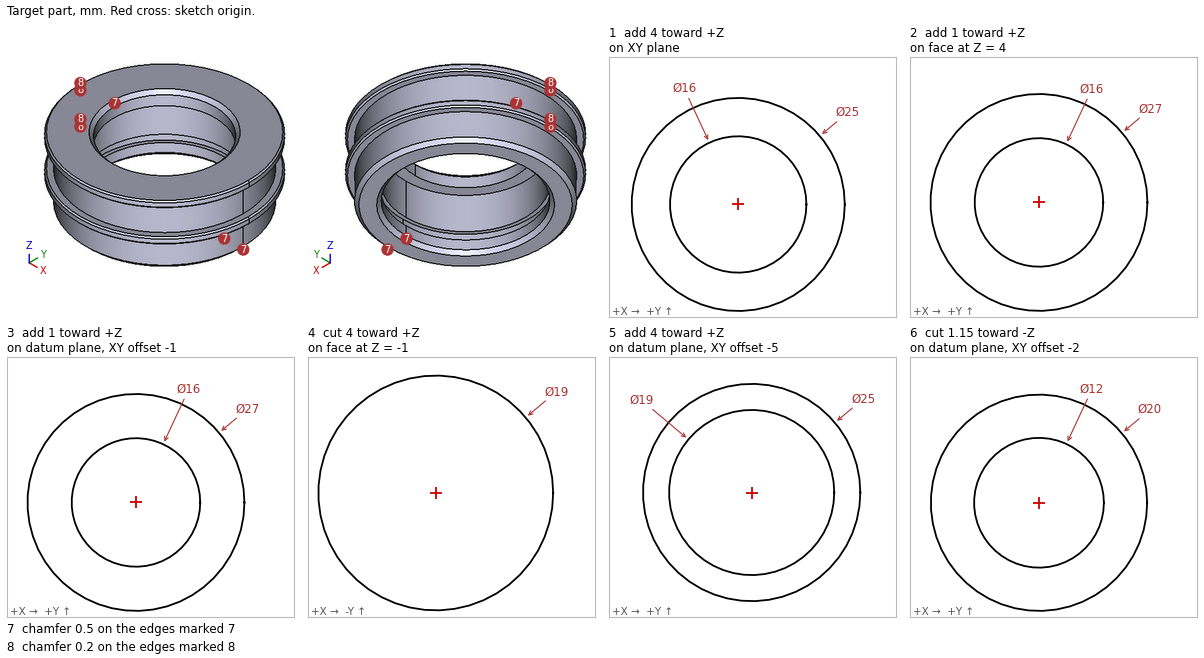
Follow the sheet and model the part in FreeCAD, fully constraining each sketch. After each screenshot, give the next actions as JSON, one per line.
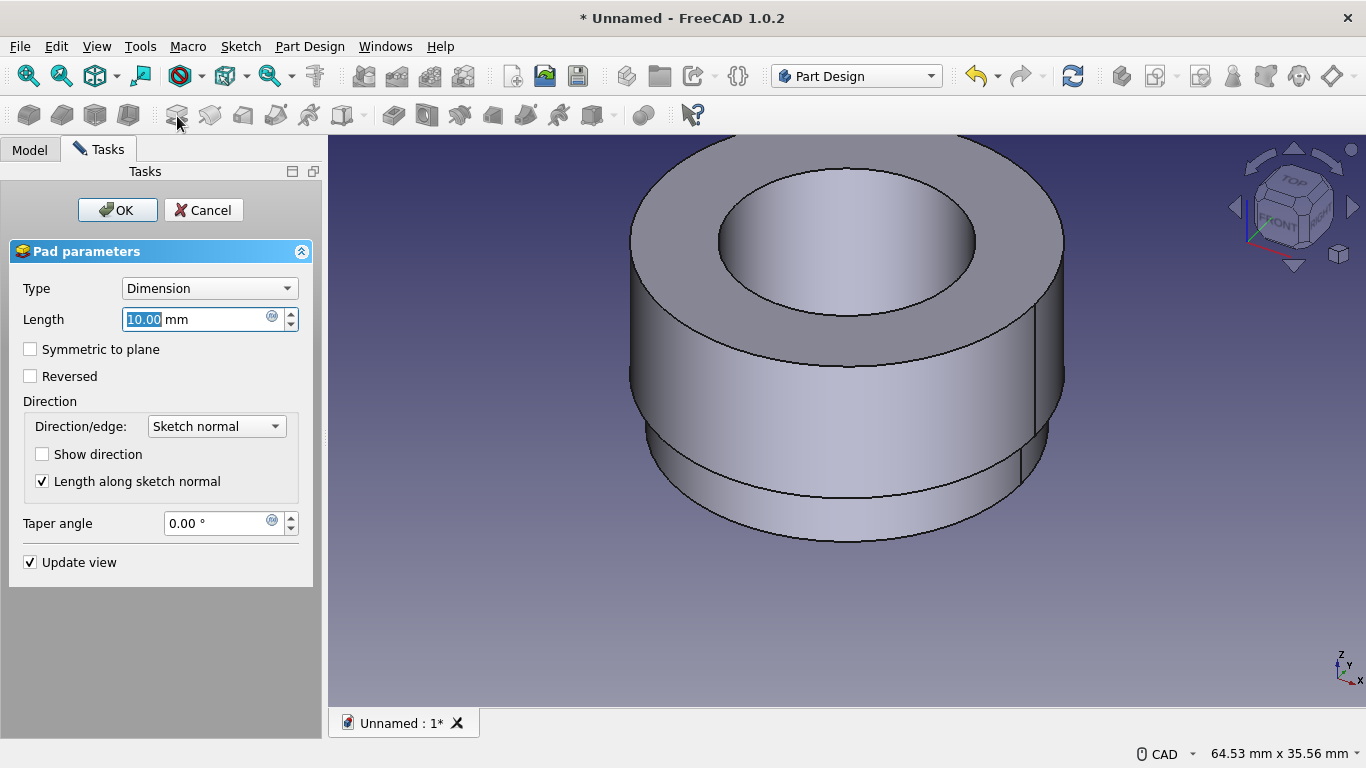
{"action": "type", "text": "1"}
{"action": "key", "text": "Tab"}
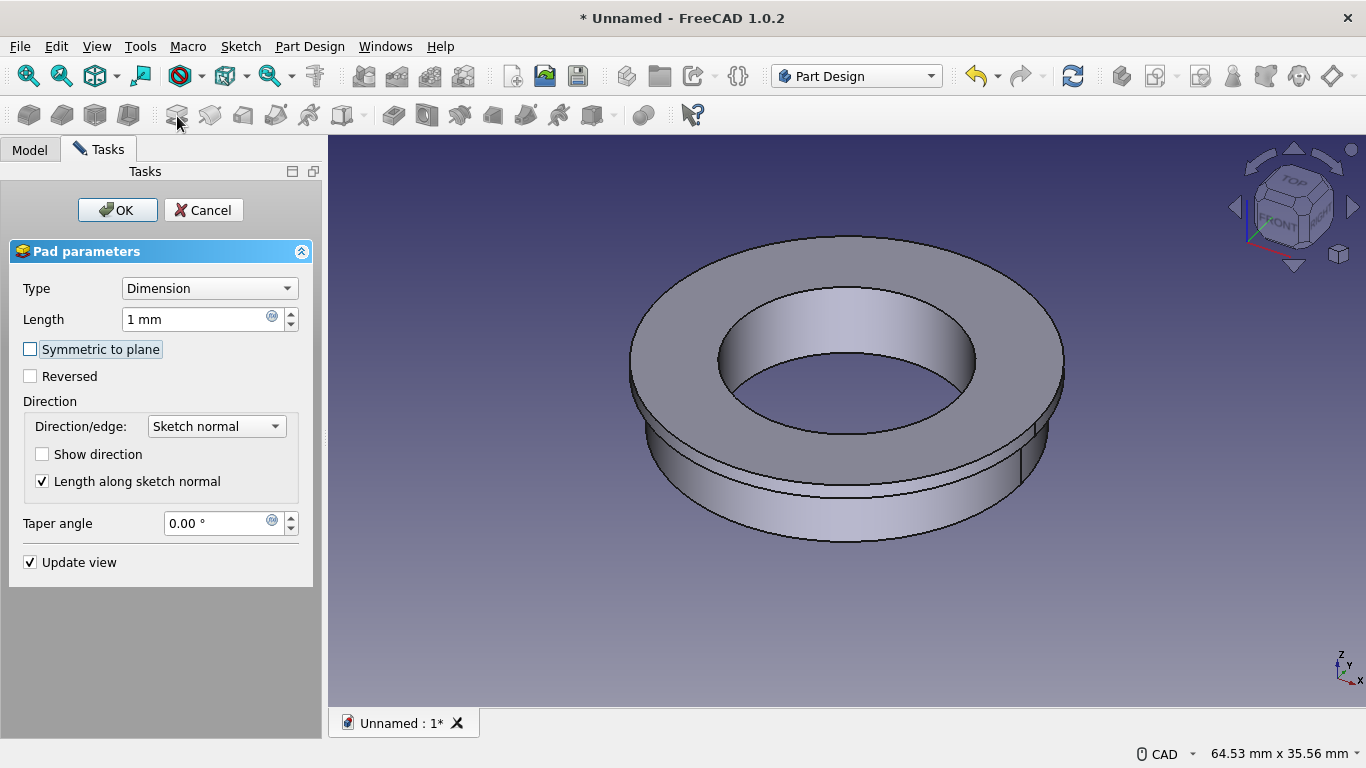
{"action": "left_click", "coordinate": [118, 210]}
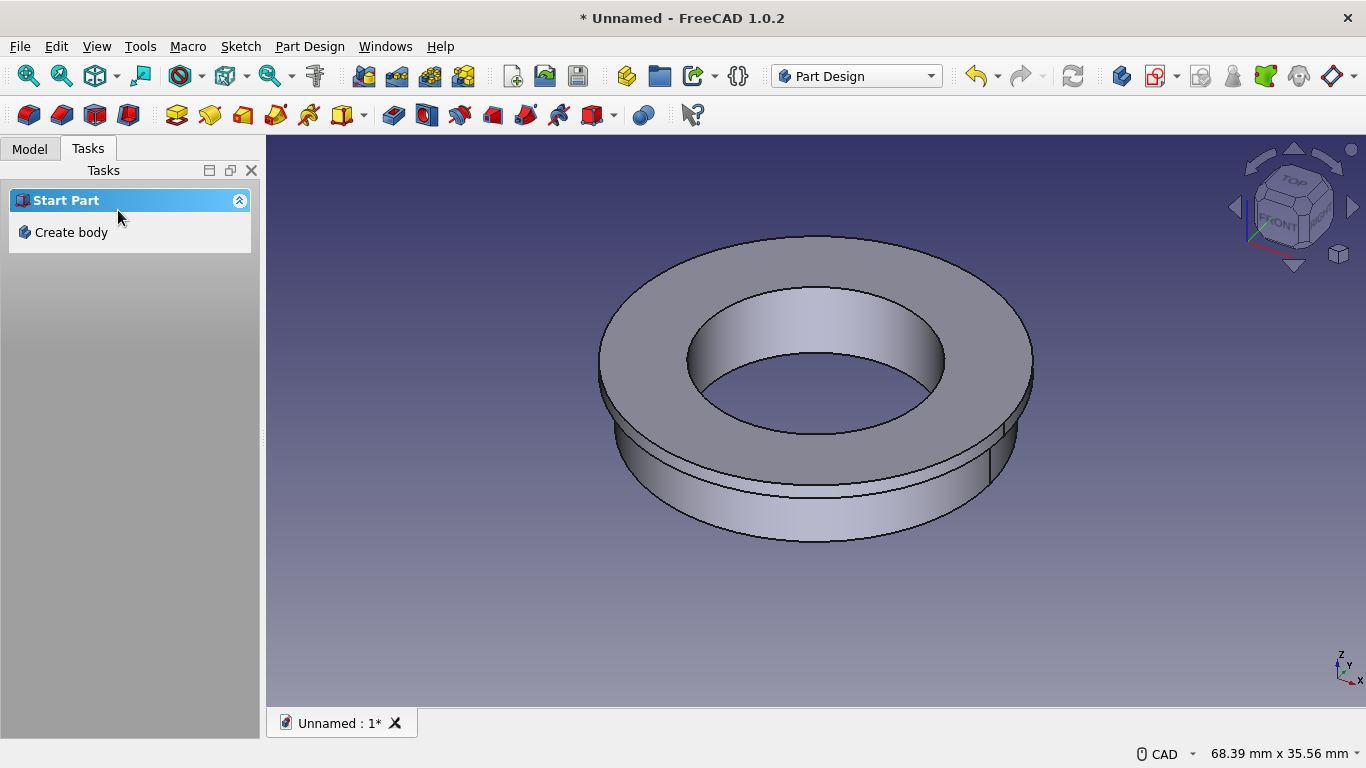
{"action": "left_click", "coordinate": [30, 148]}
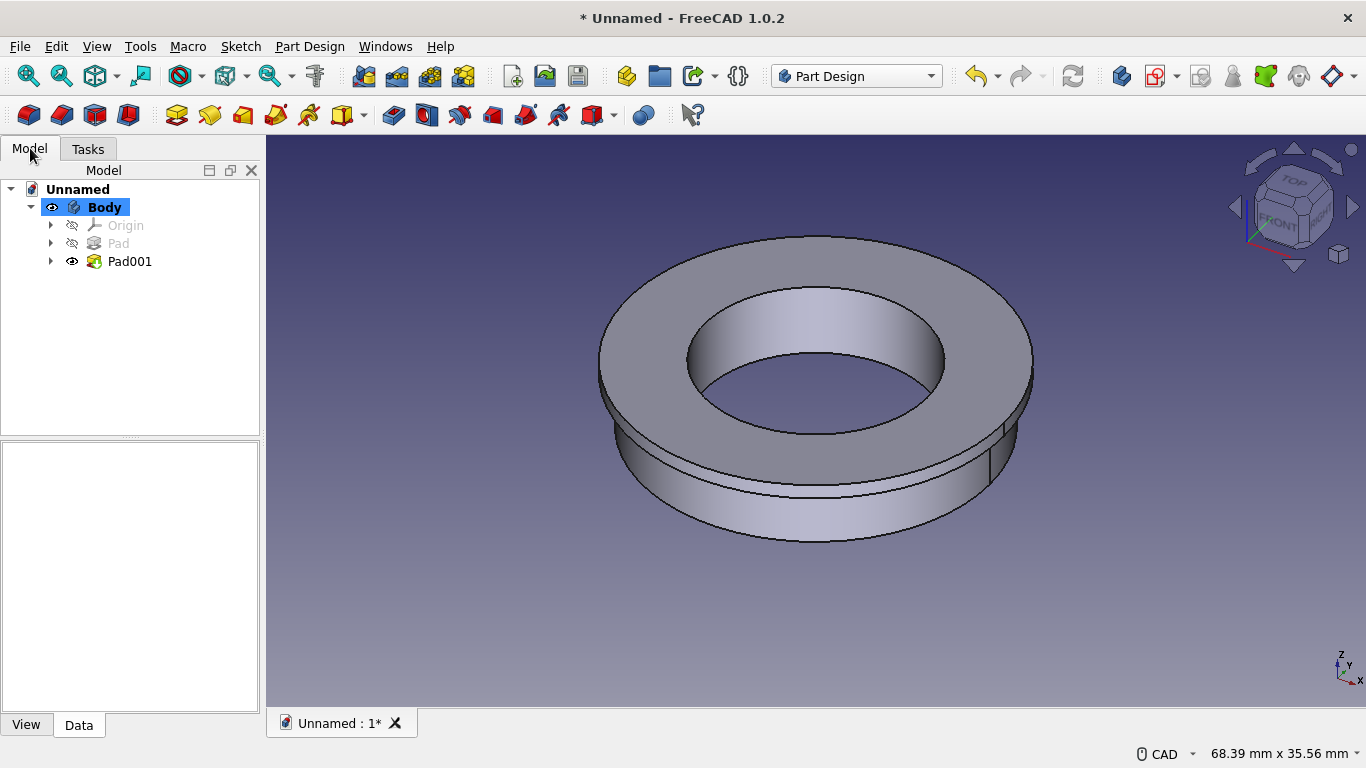
{"action": "left_click", "coordinate": [51, 225]}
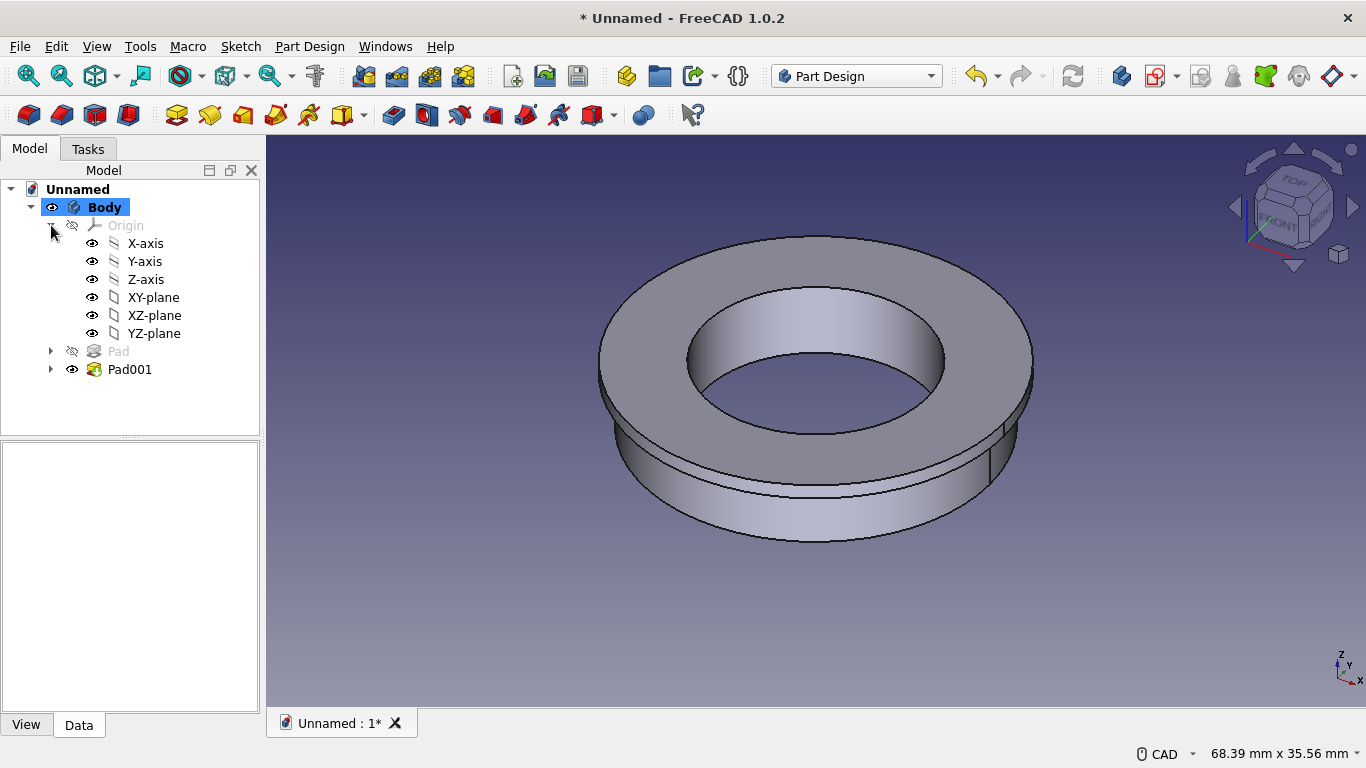
{"action": "left_click", "coordinate": [137, 297]}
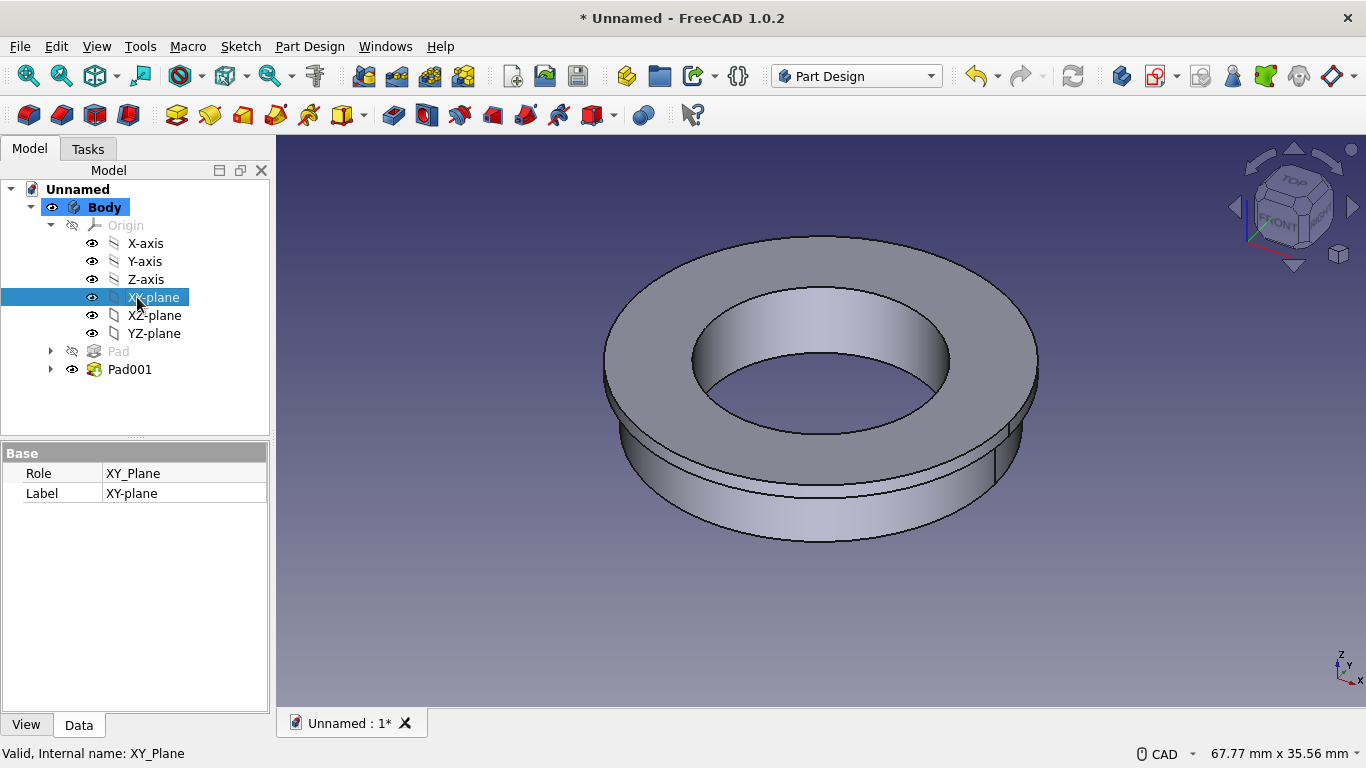
{"action": "left_click", "coordinate": [1332, 76]}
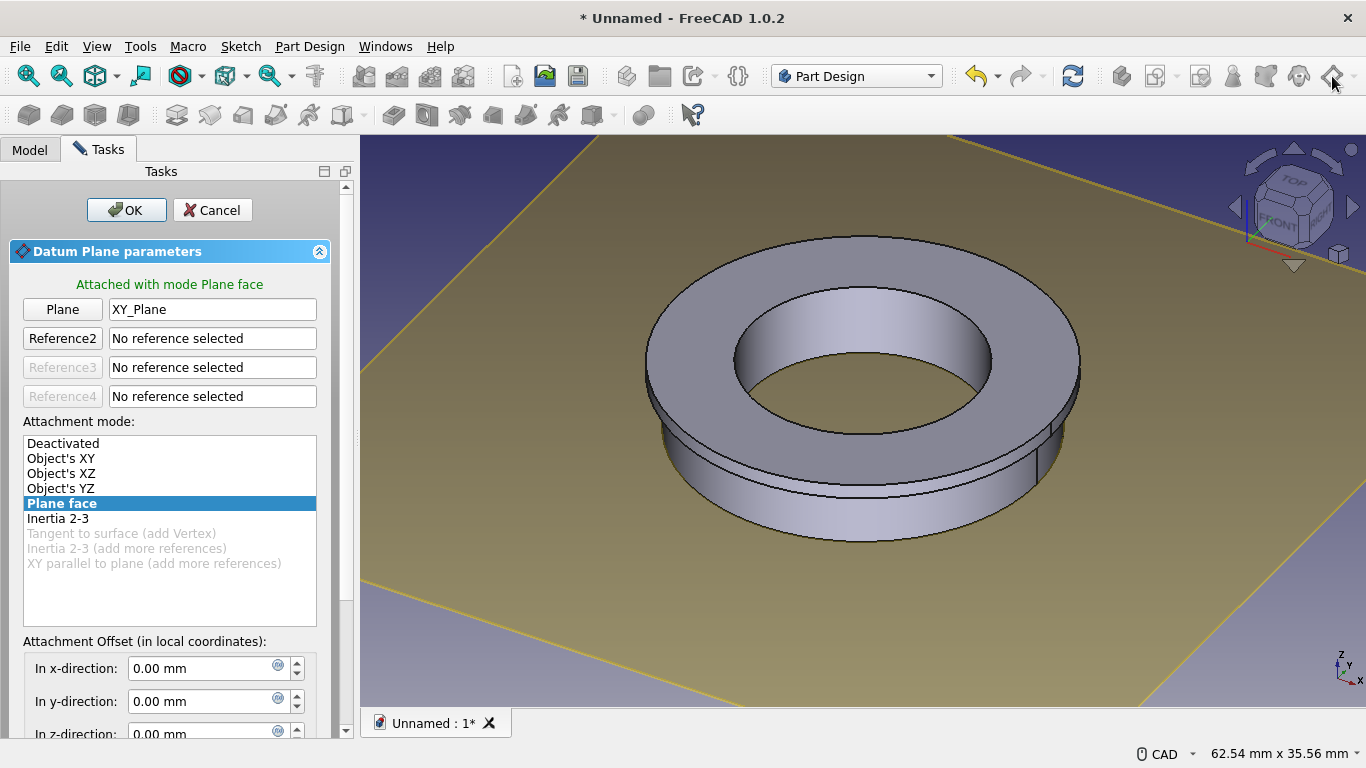
{"action": "scroll", "coordinate": [346, 460], "scroll_direction": "down", "scroll_amount": 2}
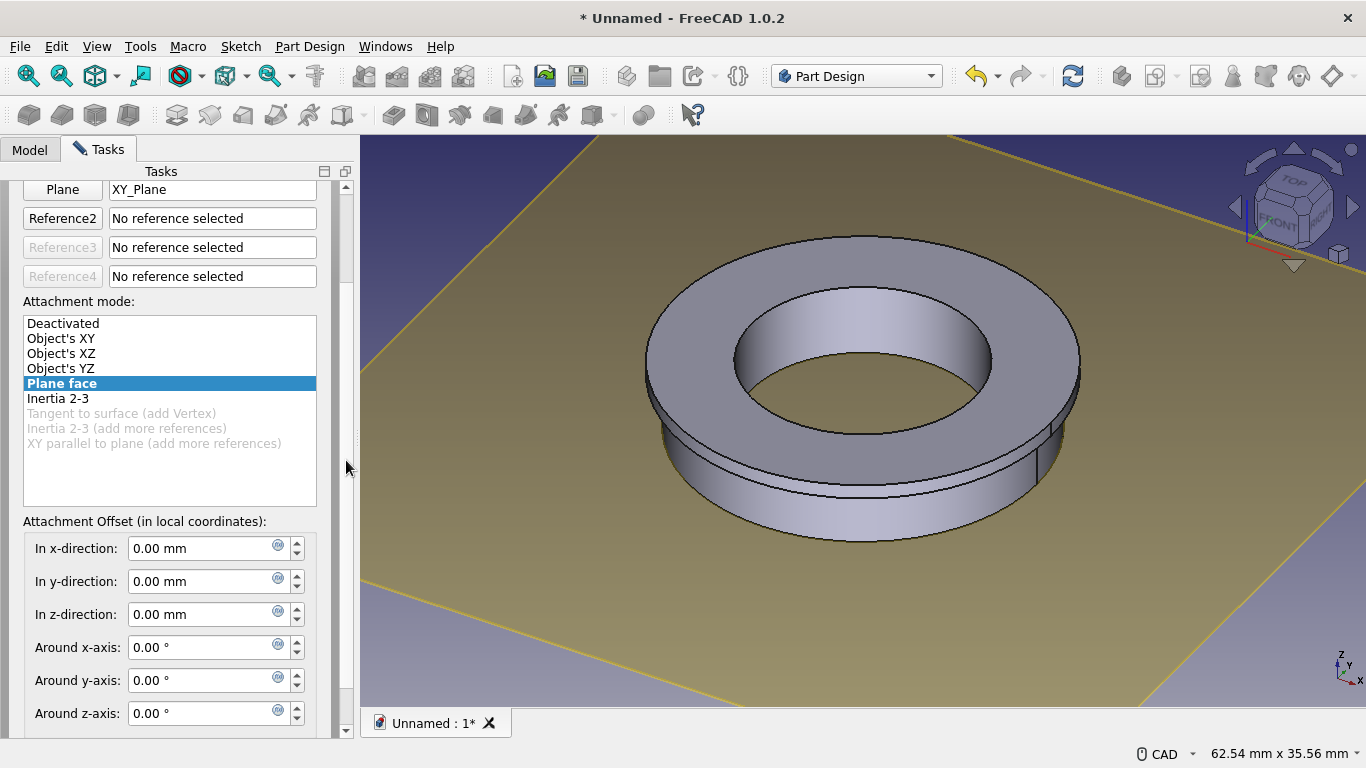
{"action": "triple_click", "coordinate": [210, 614]}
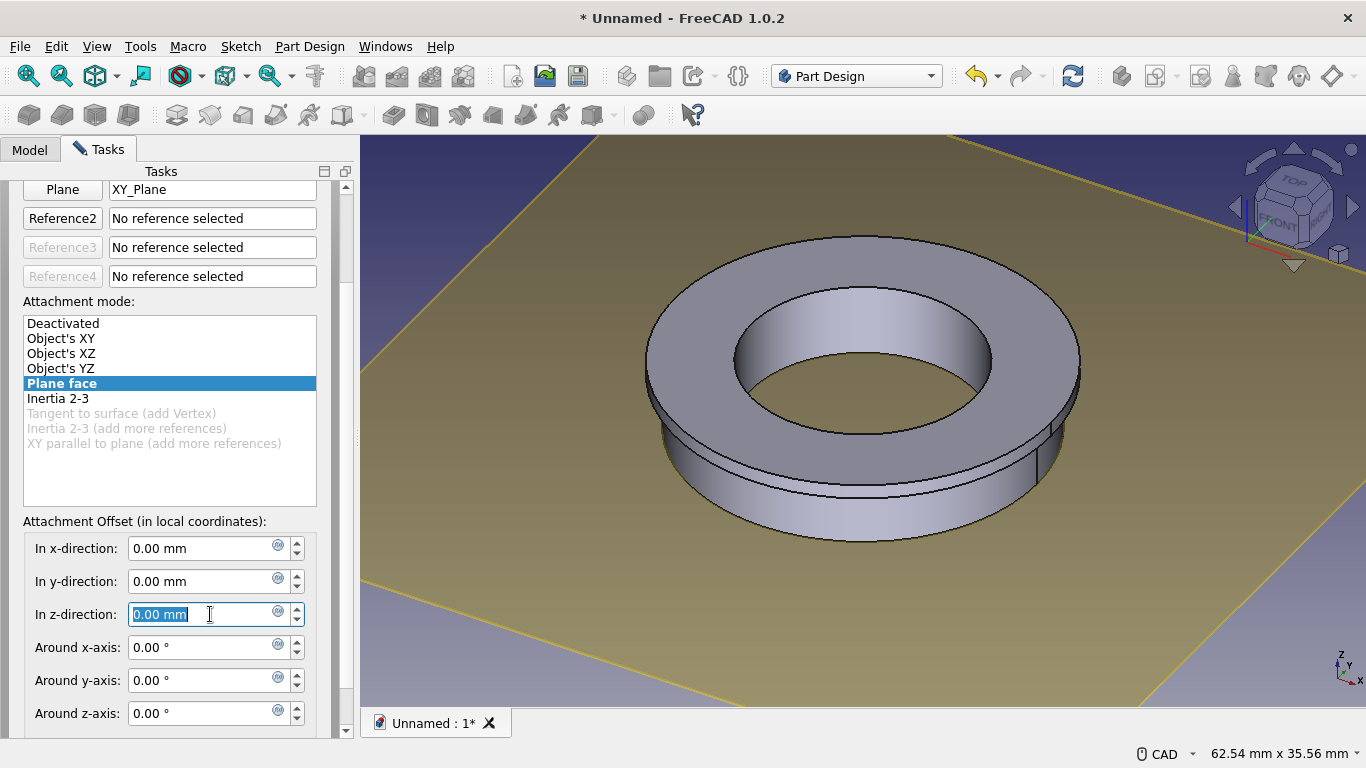
{"action": "type", "text": "-1"}
{"action": "key", "text": "Tab"}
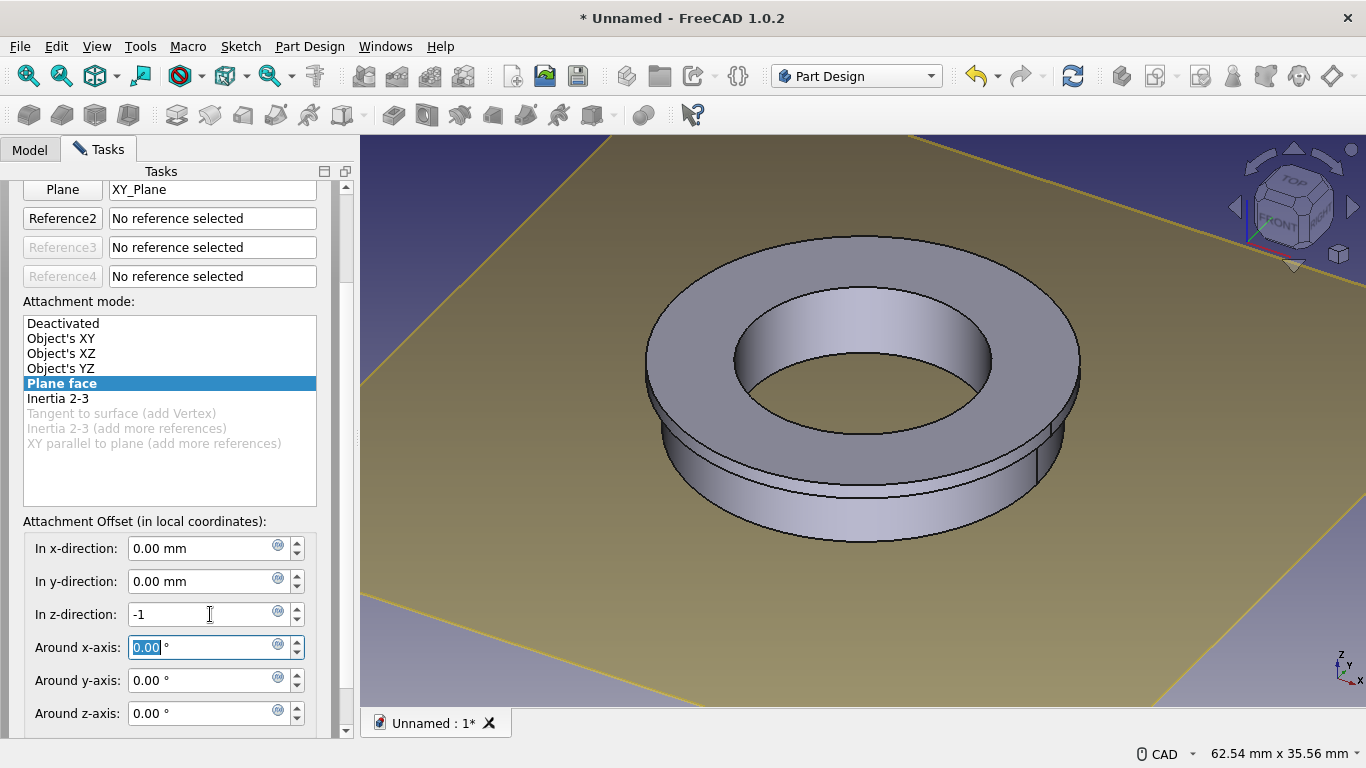
{"action": "scroll", "coordinate": [346, 460], "scroll_direction": "up", "scroll_amount": 3}